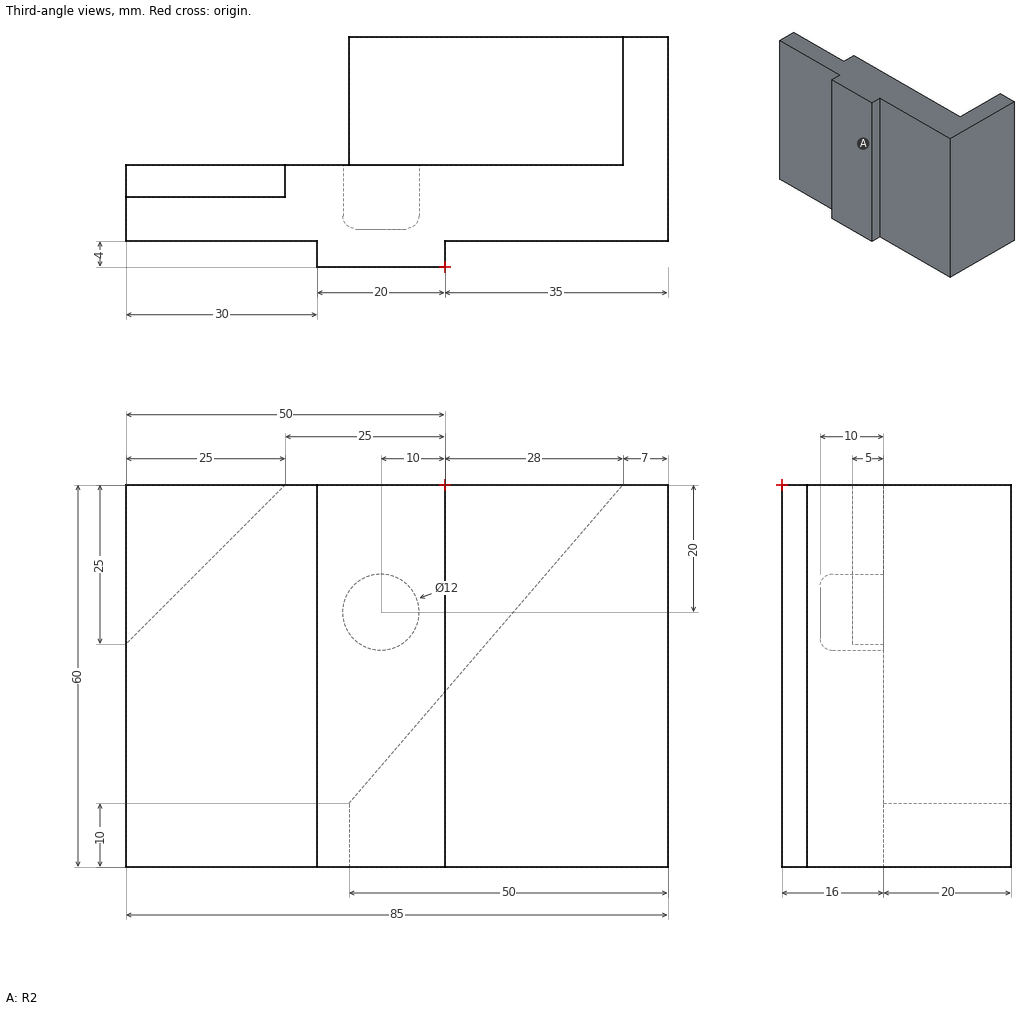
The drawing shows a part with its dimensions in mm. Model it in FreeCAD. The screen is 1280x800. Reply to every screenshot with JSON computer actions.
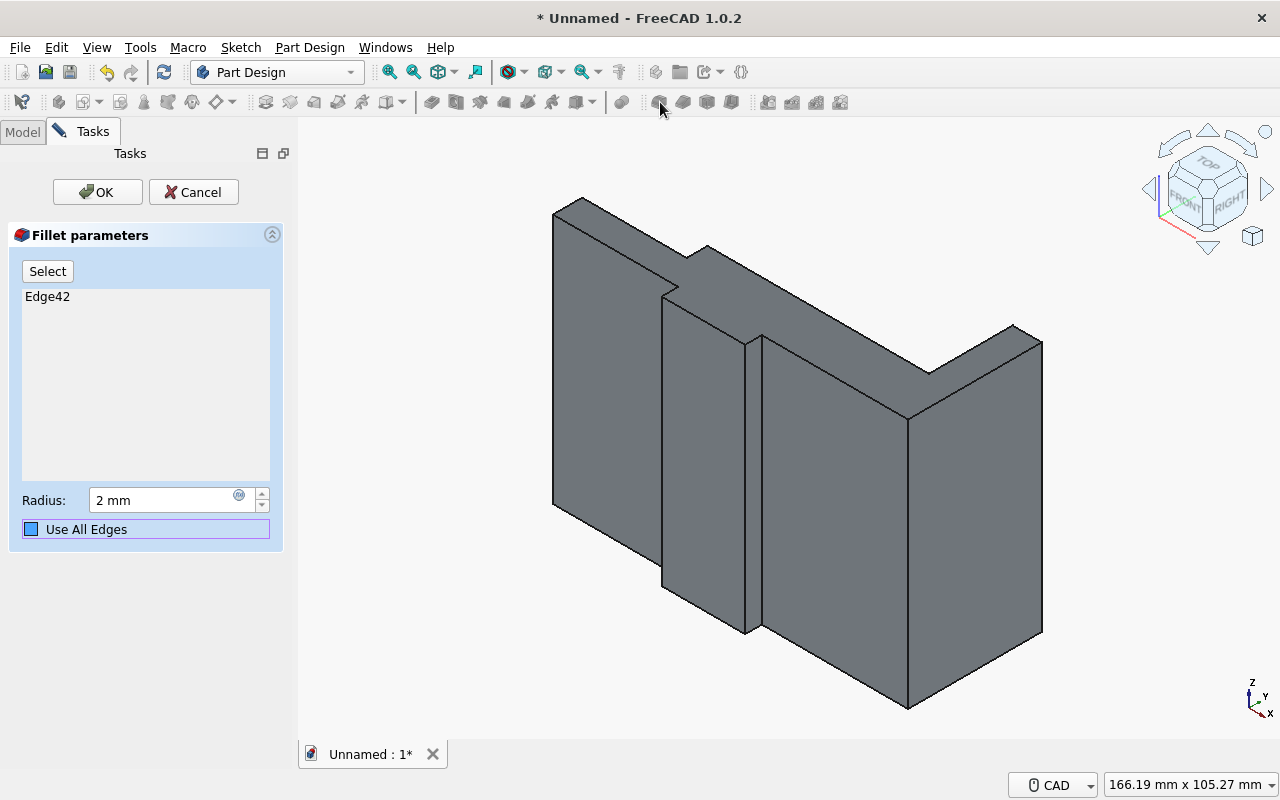
{"action": "left_click", "coordinate": [98, 192]}